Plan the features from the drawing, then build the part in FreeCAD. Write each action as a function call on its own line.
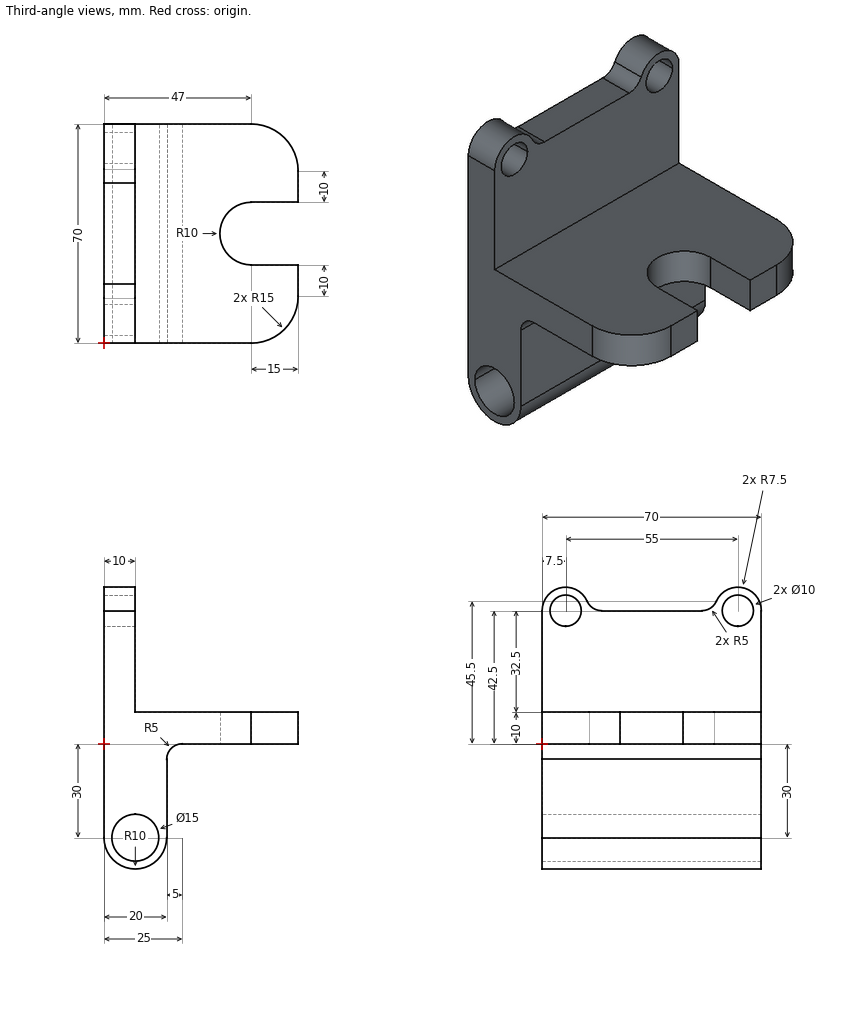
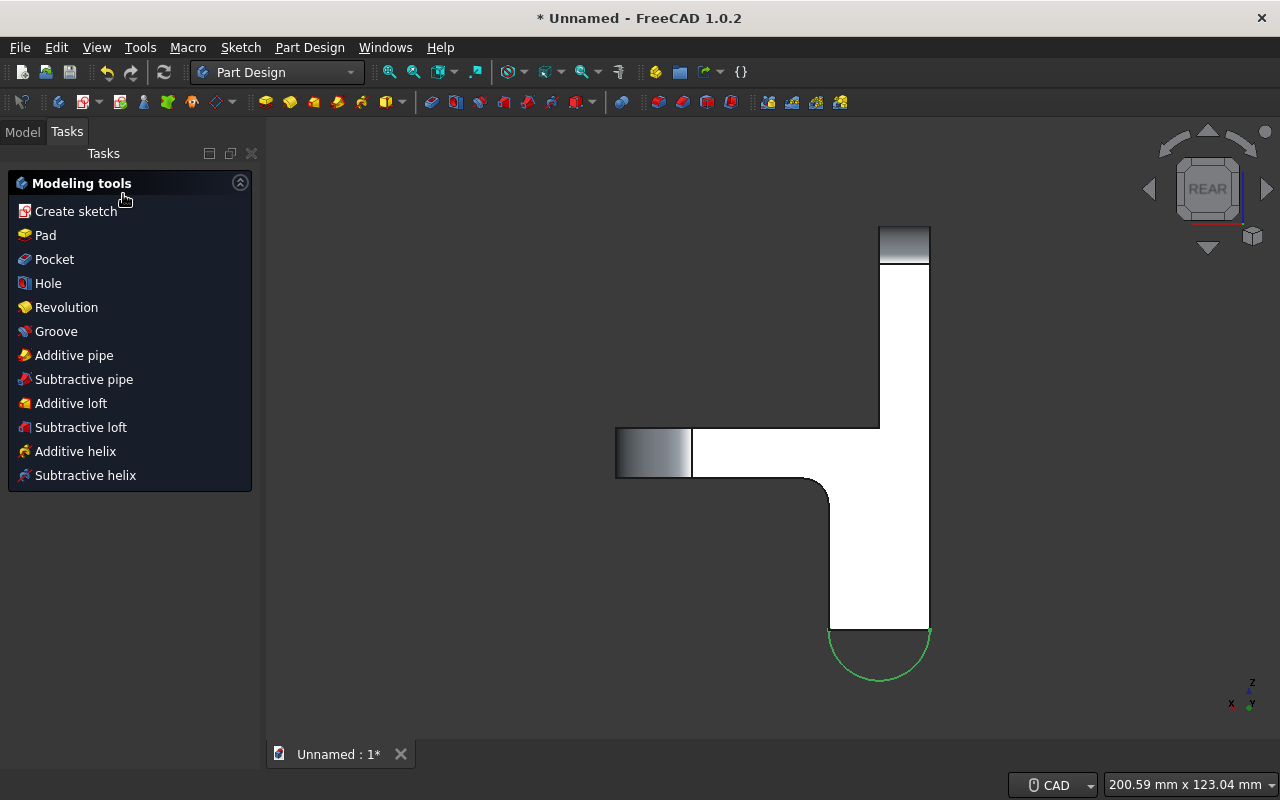
click(266, 102)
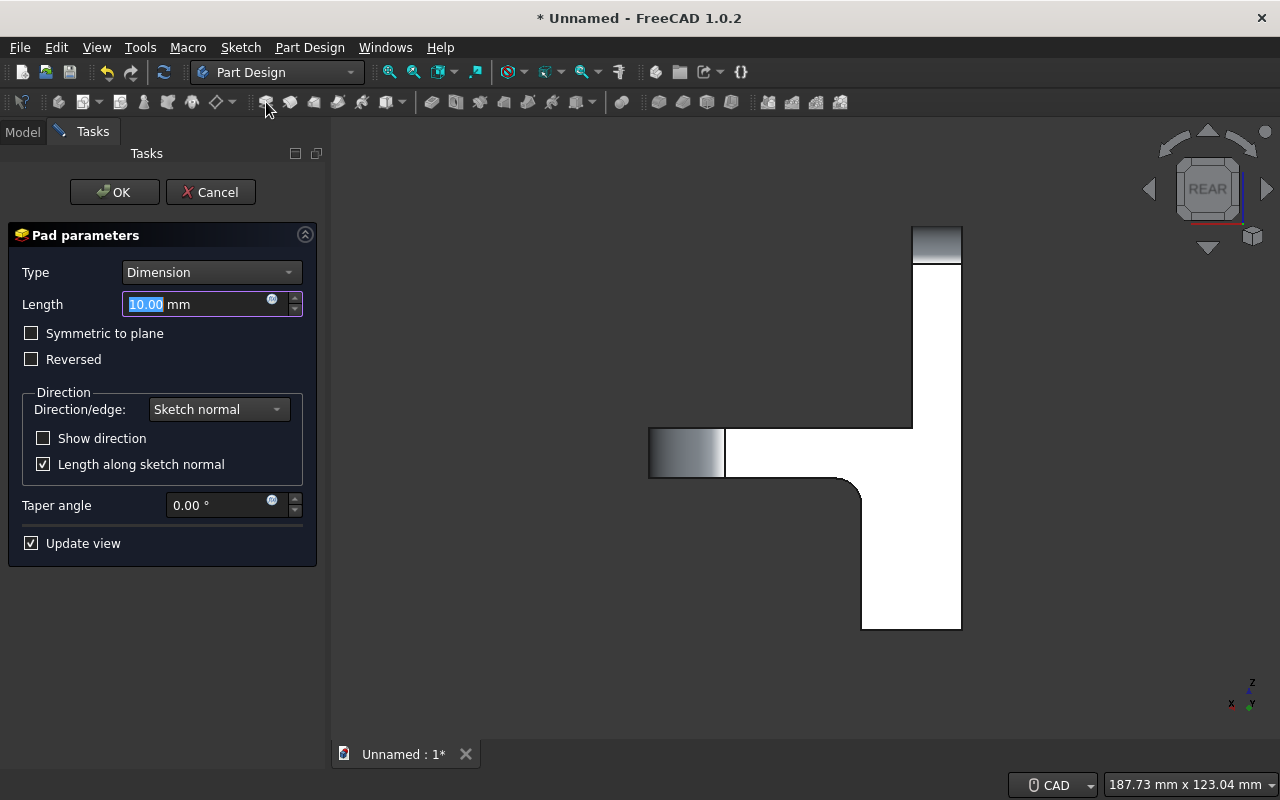
text(70)
key(Tab)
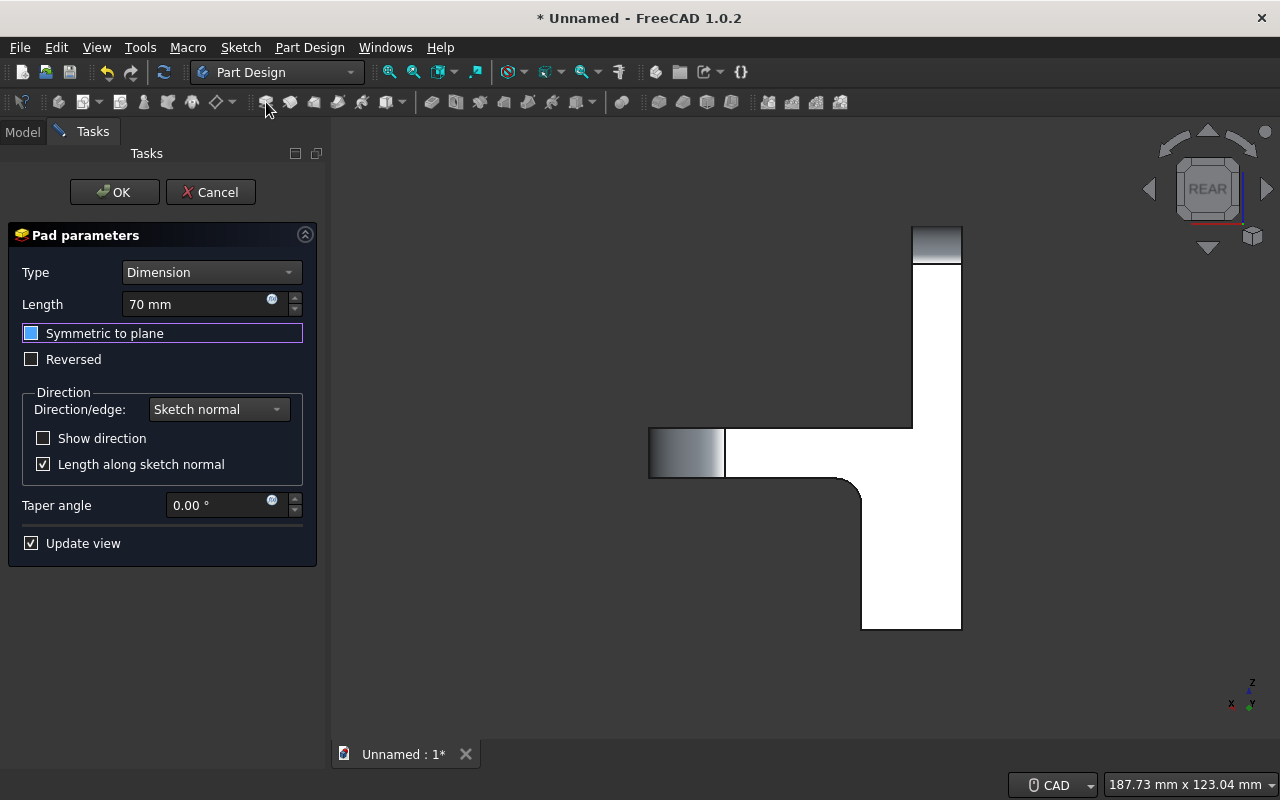
click(30, 359)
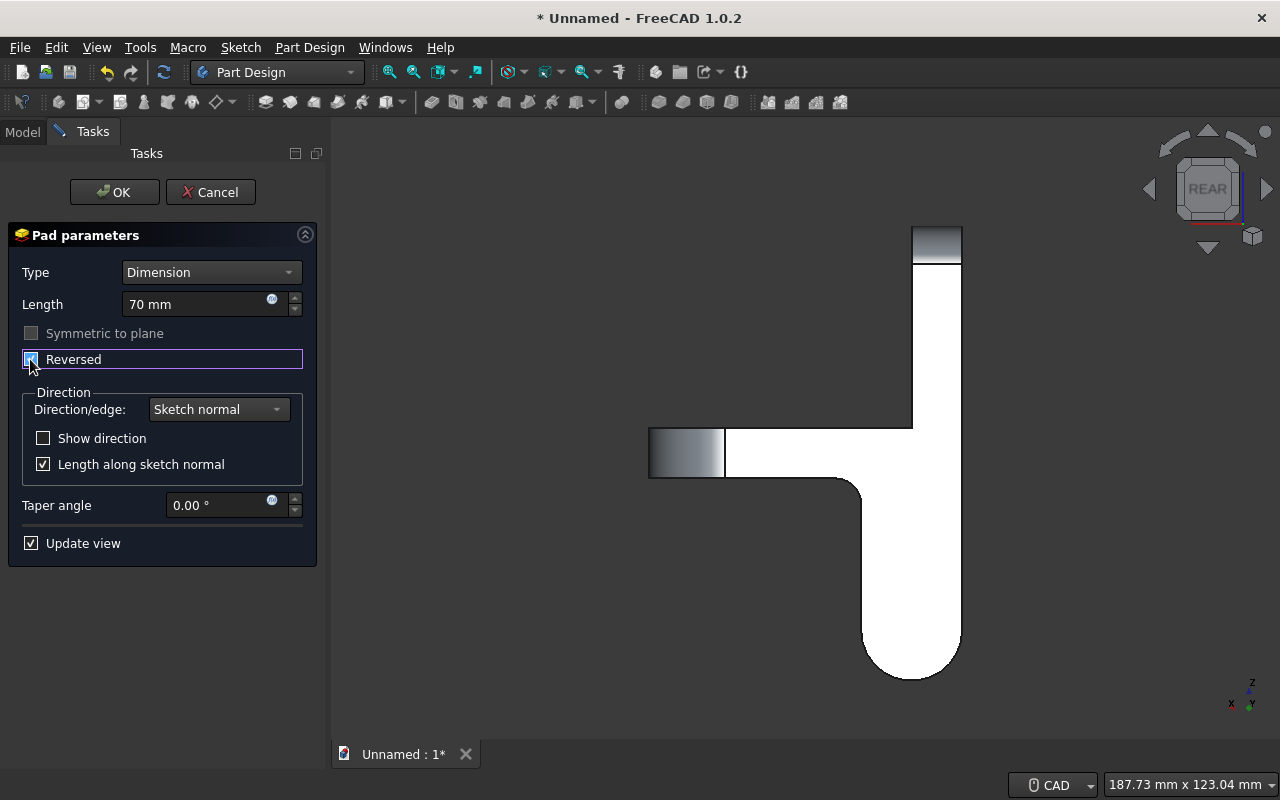
click(115, 192)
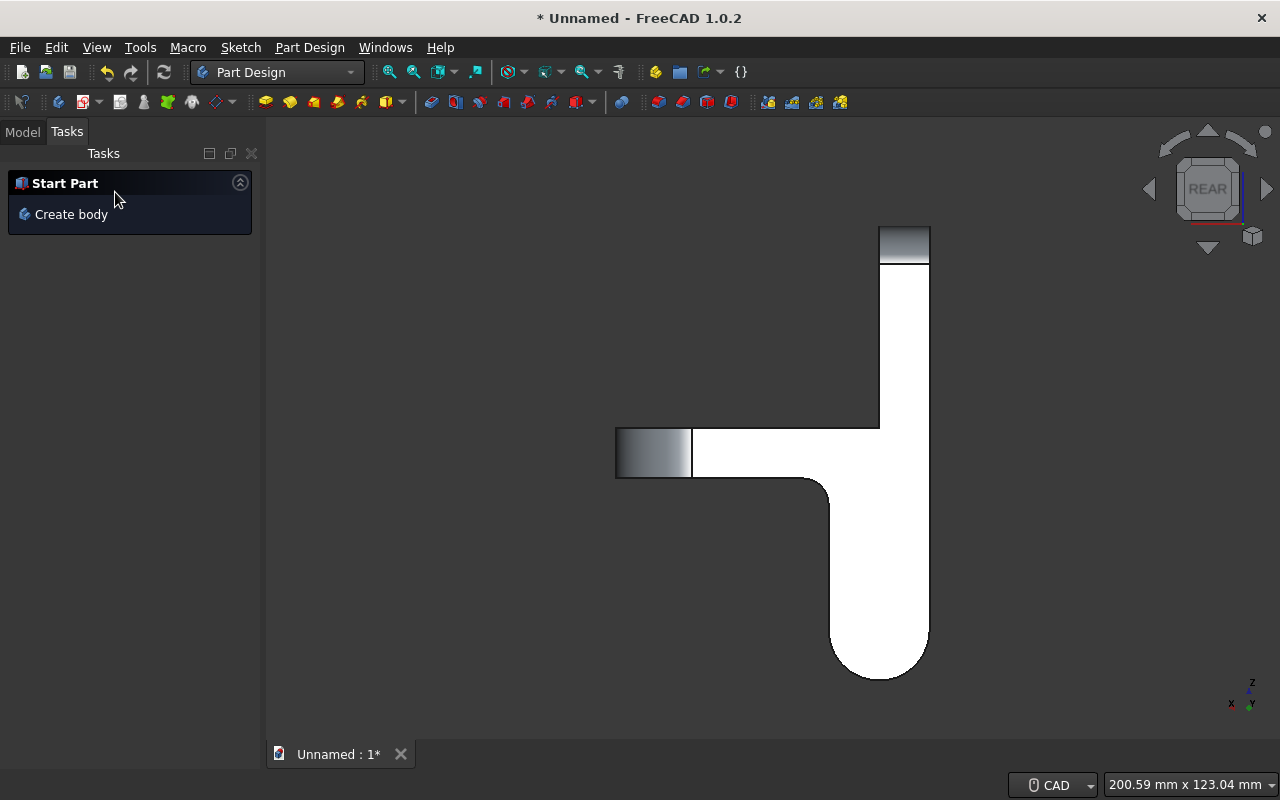
click(879, 531)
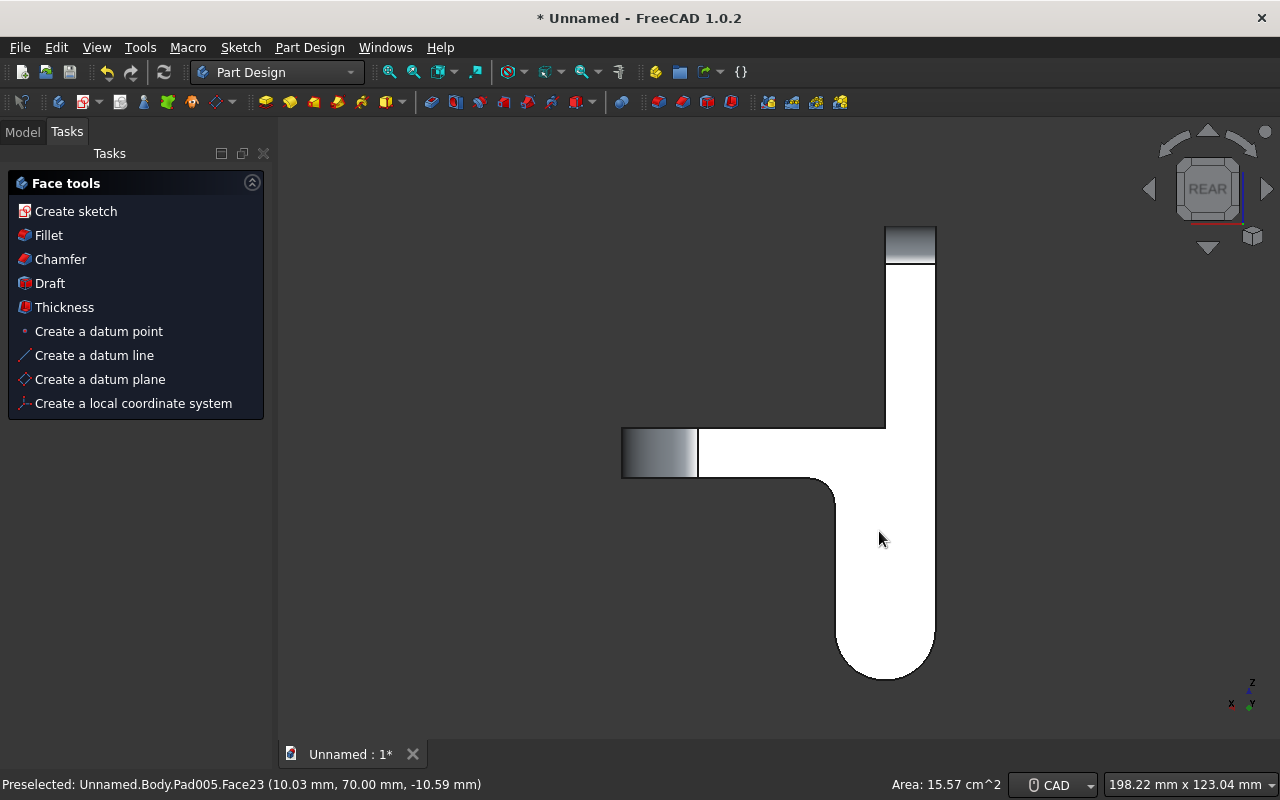
click(84, 102)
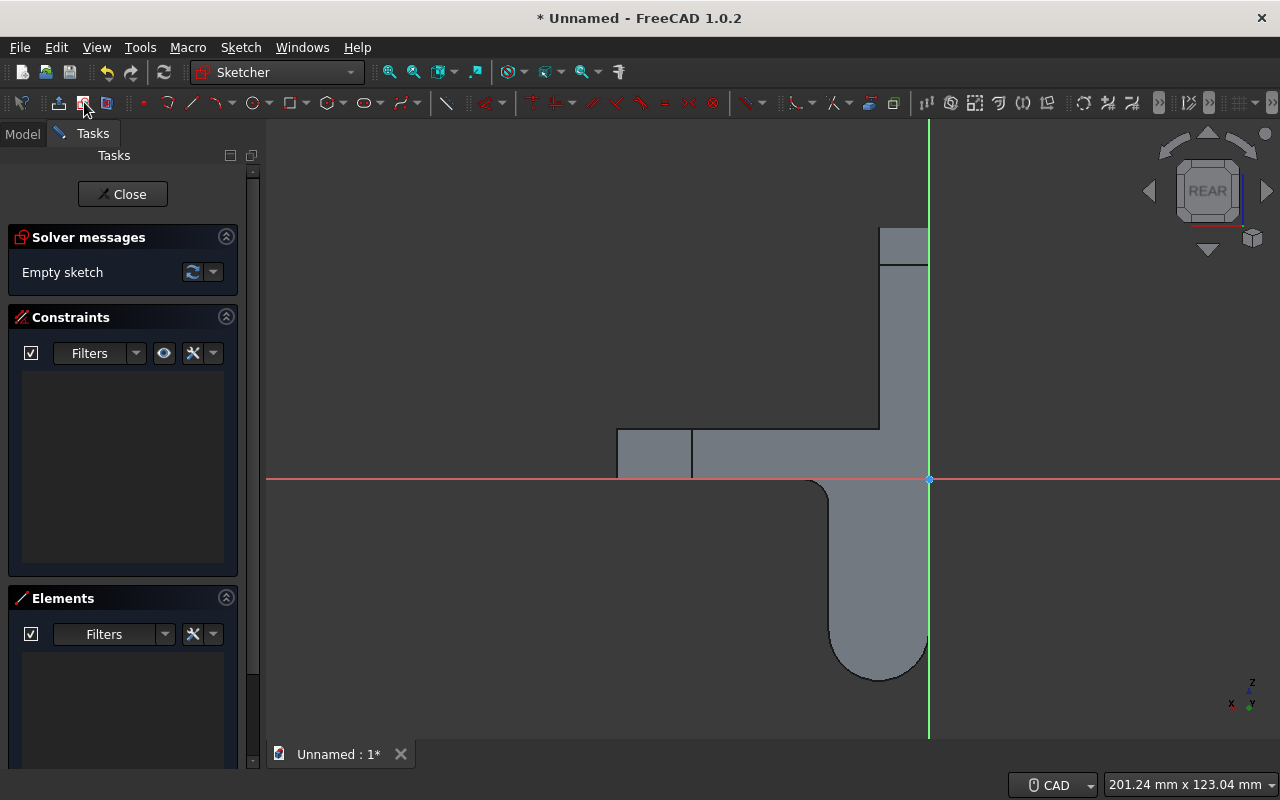
scroll(923, 681, up, 8)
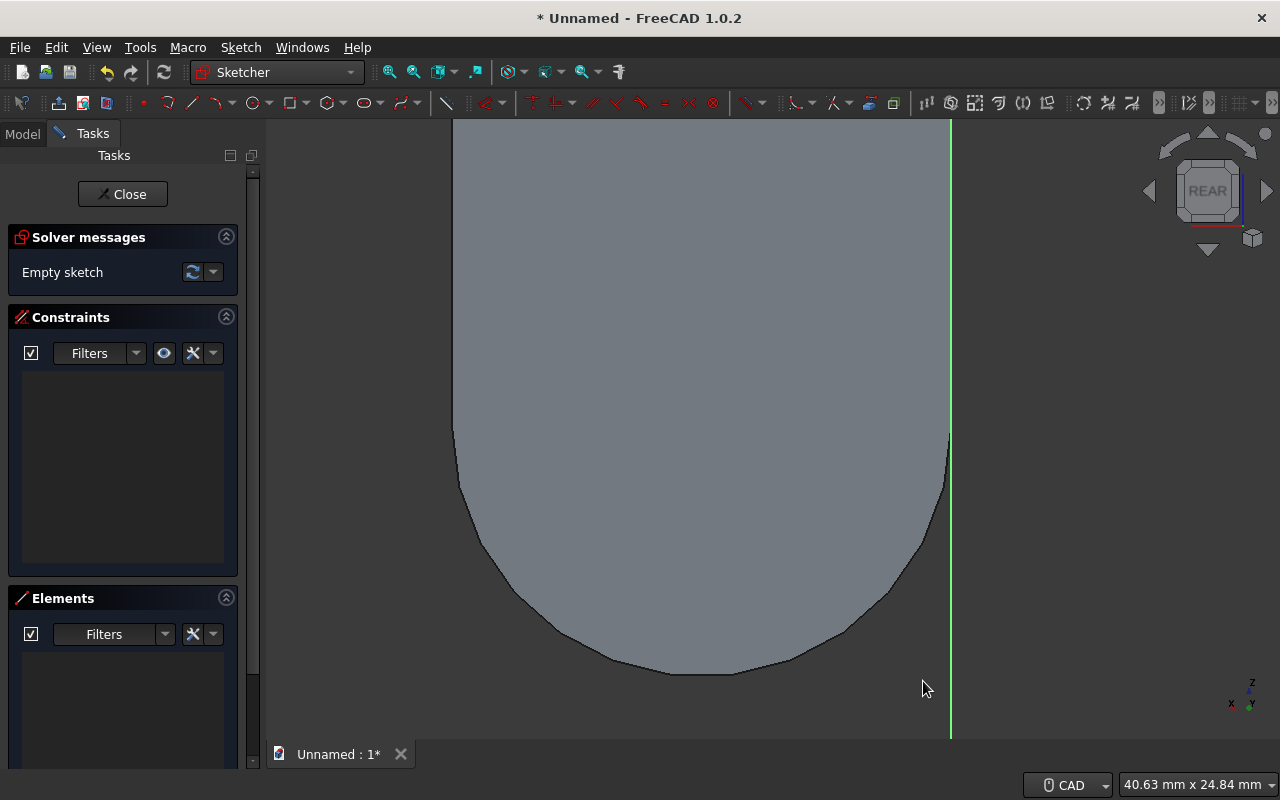
click(254, 104)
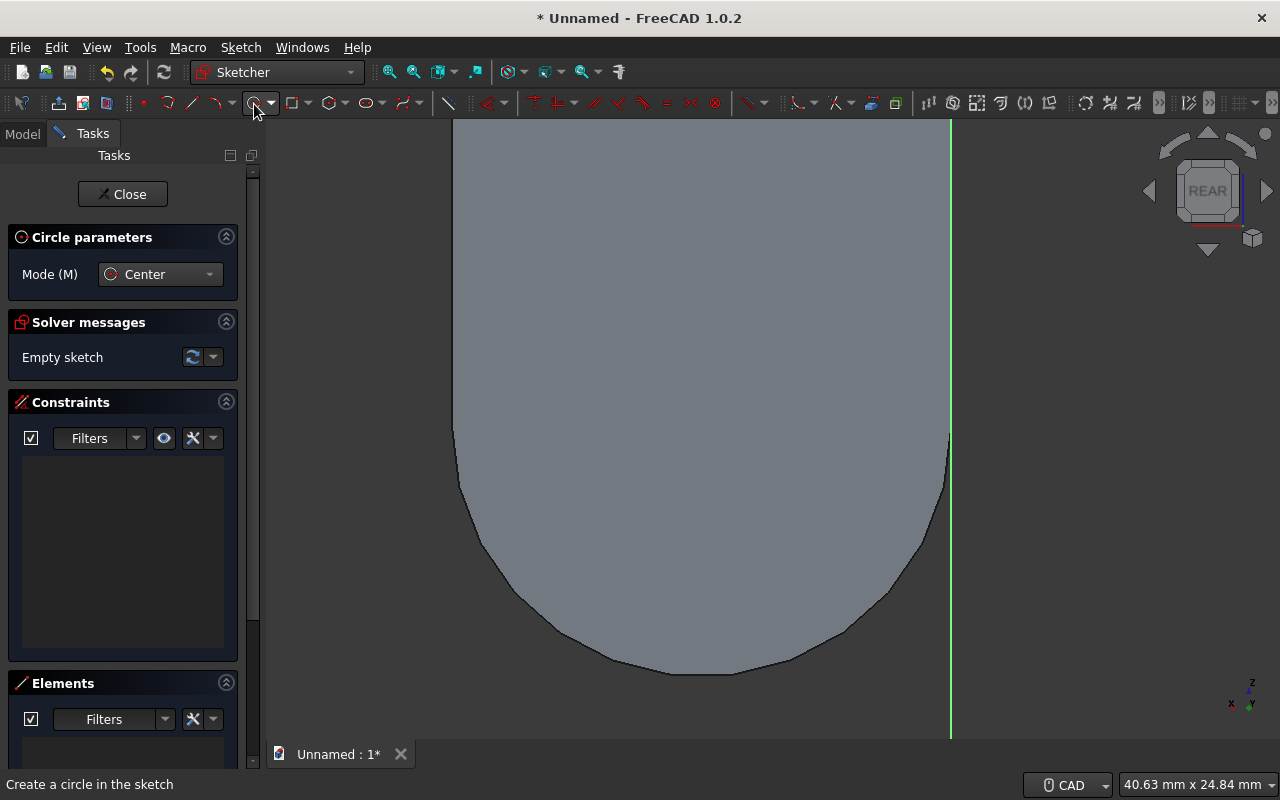
click(702, 427)
click(834, 295)
key(Escape)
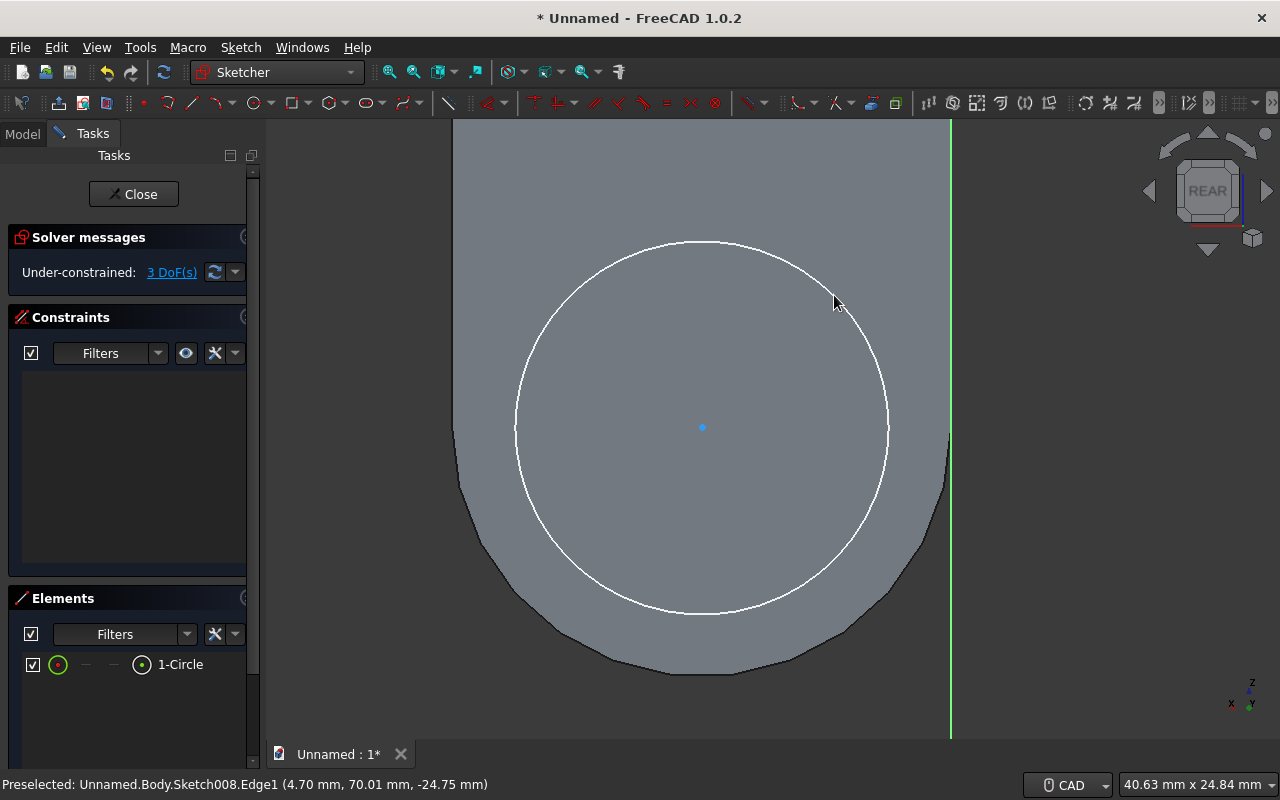
click(488, 104)